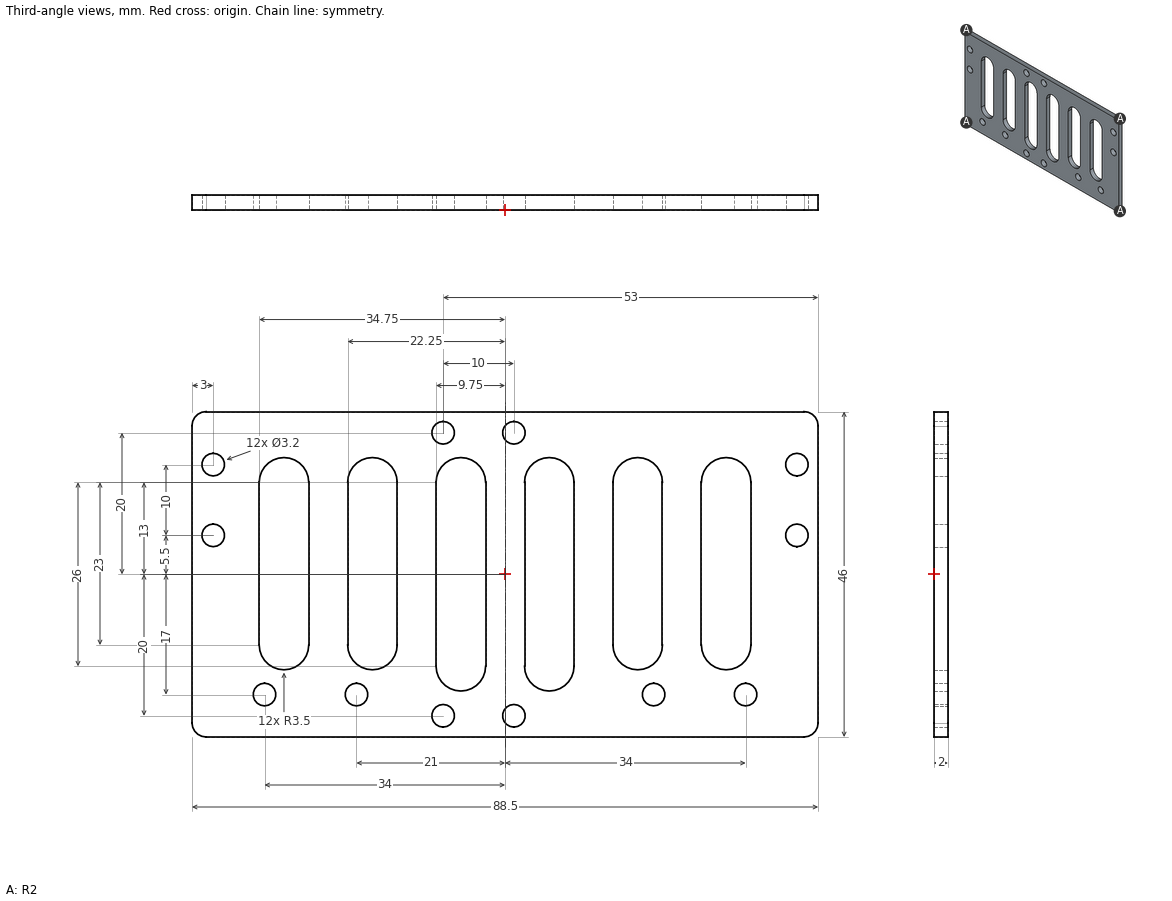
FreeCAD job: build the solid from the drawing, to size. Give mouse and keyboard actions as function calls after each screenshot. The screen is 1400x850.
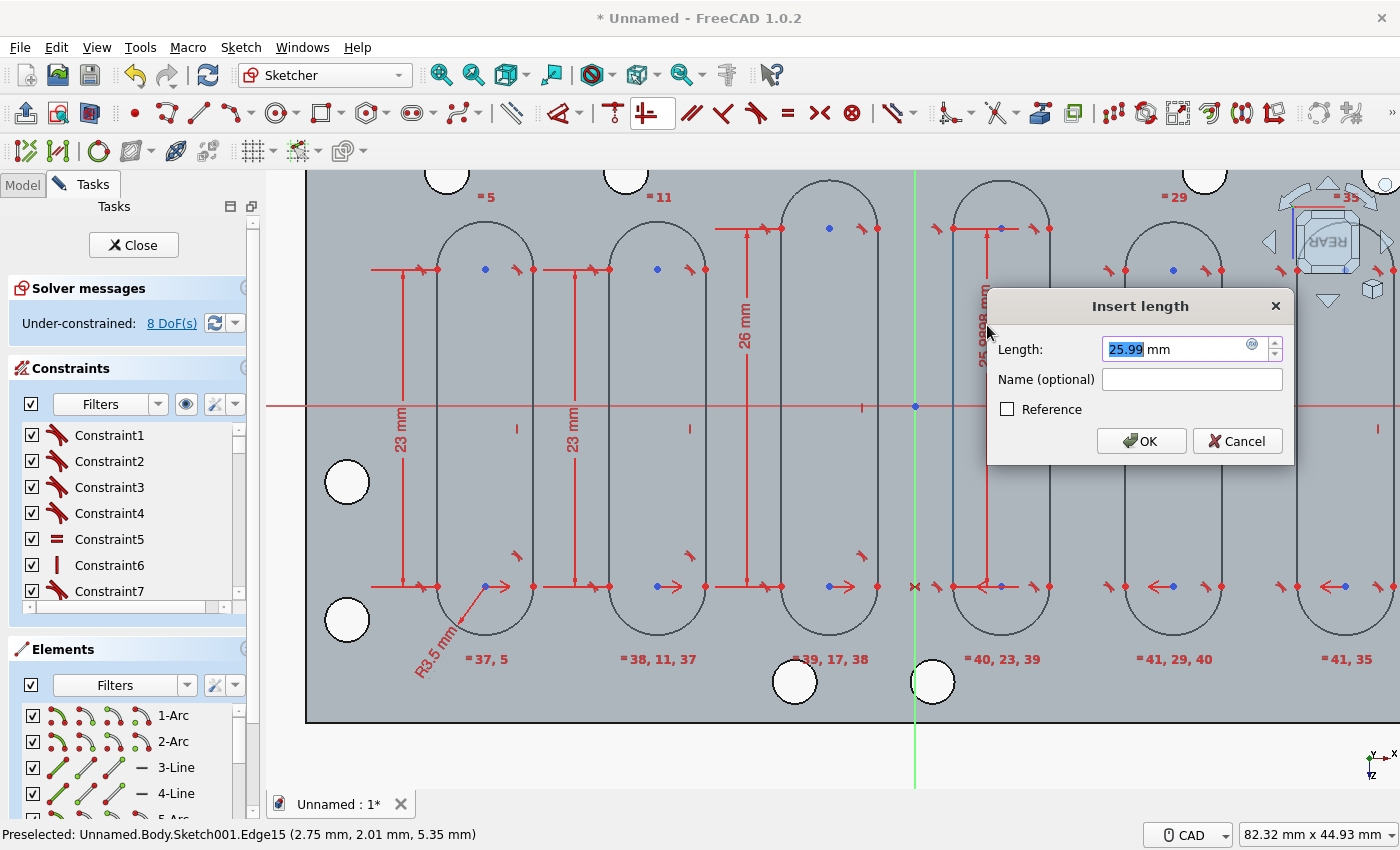
text(26)
key(Return)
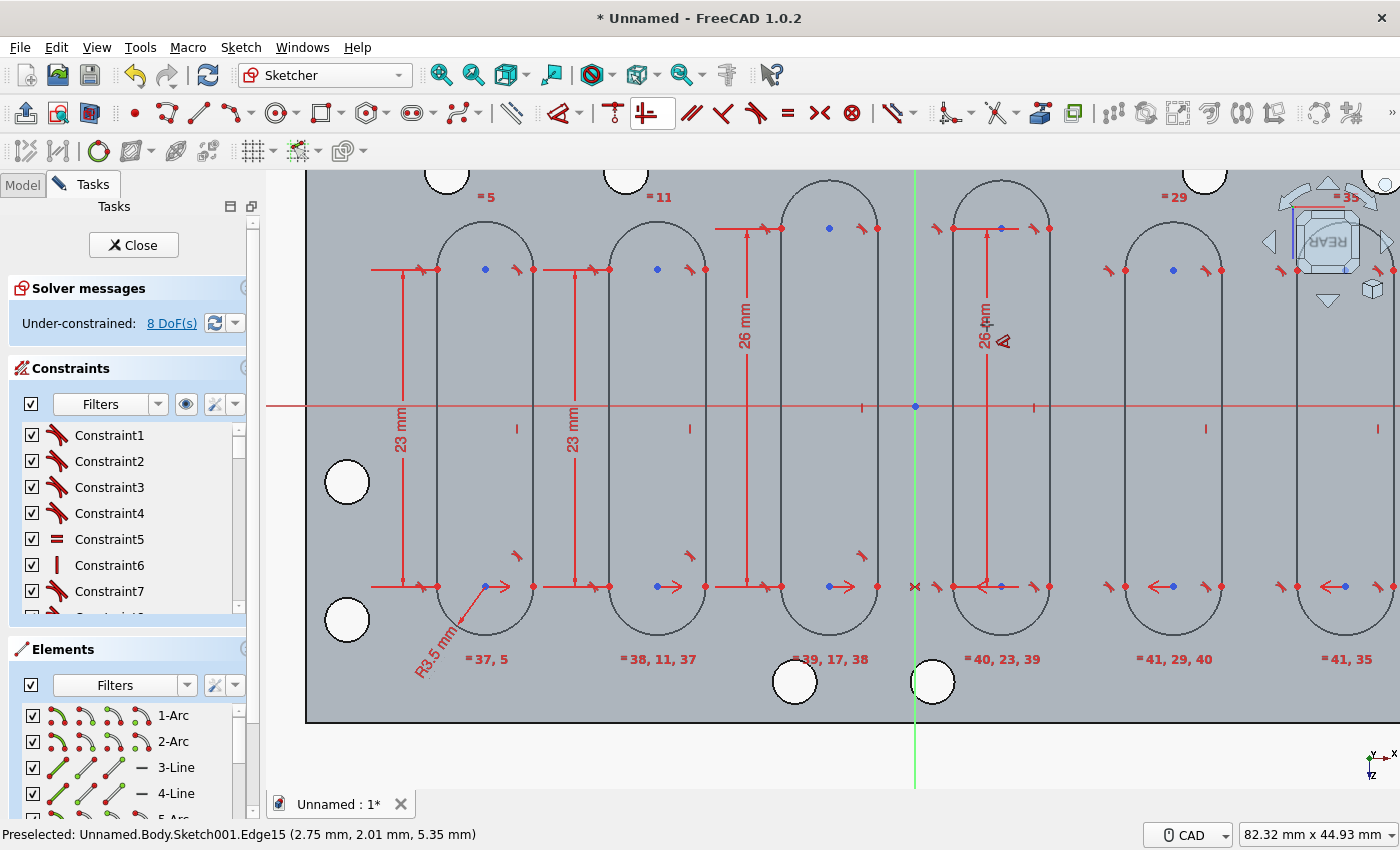
click(1125, 492)
click(1159, 429)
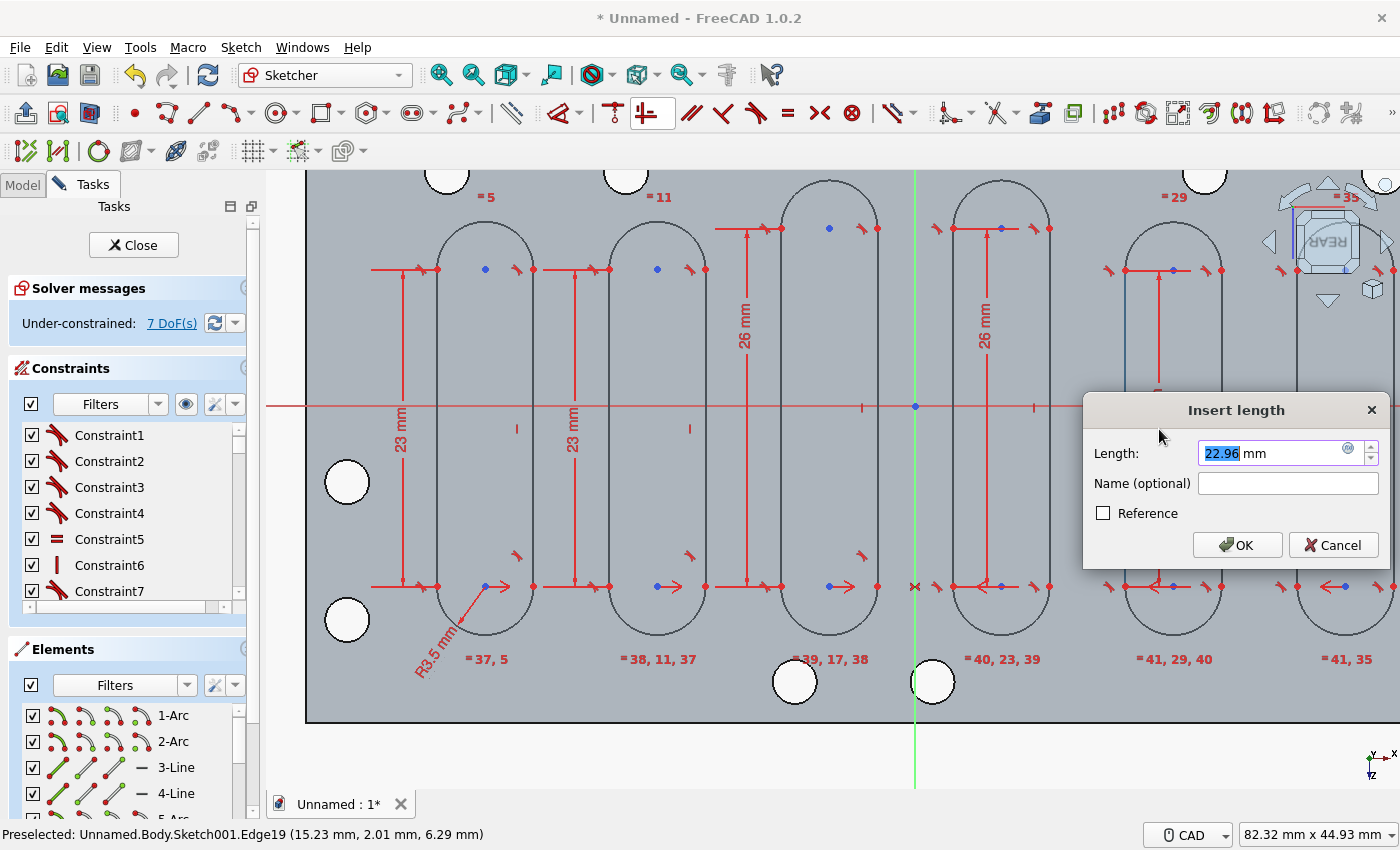
text(23)
key(Return)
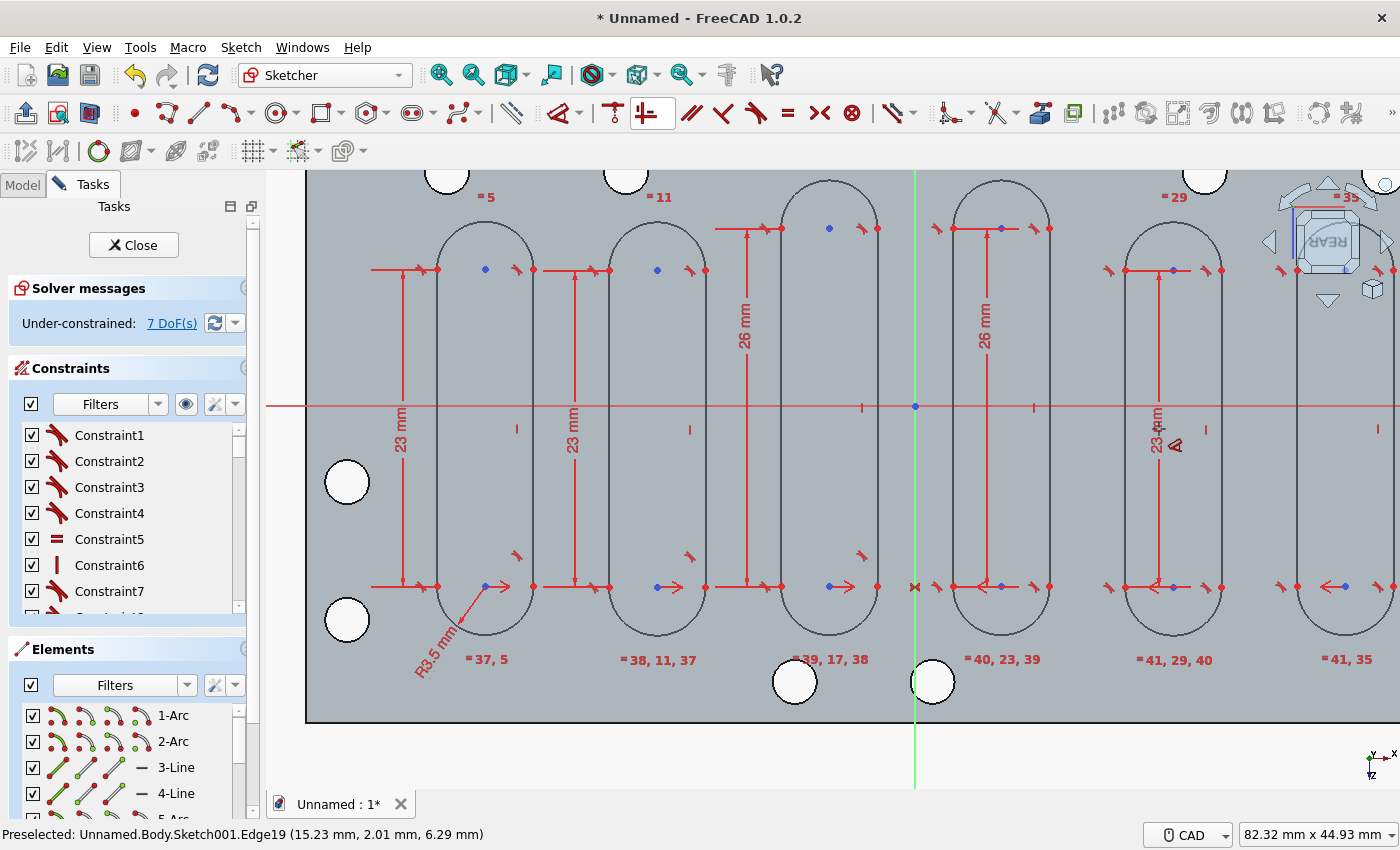
scroll(458, 628, down, 2)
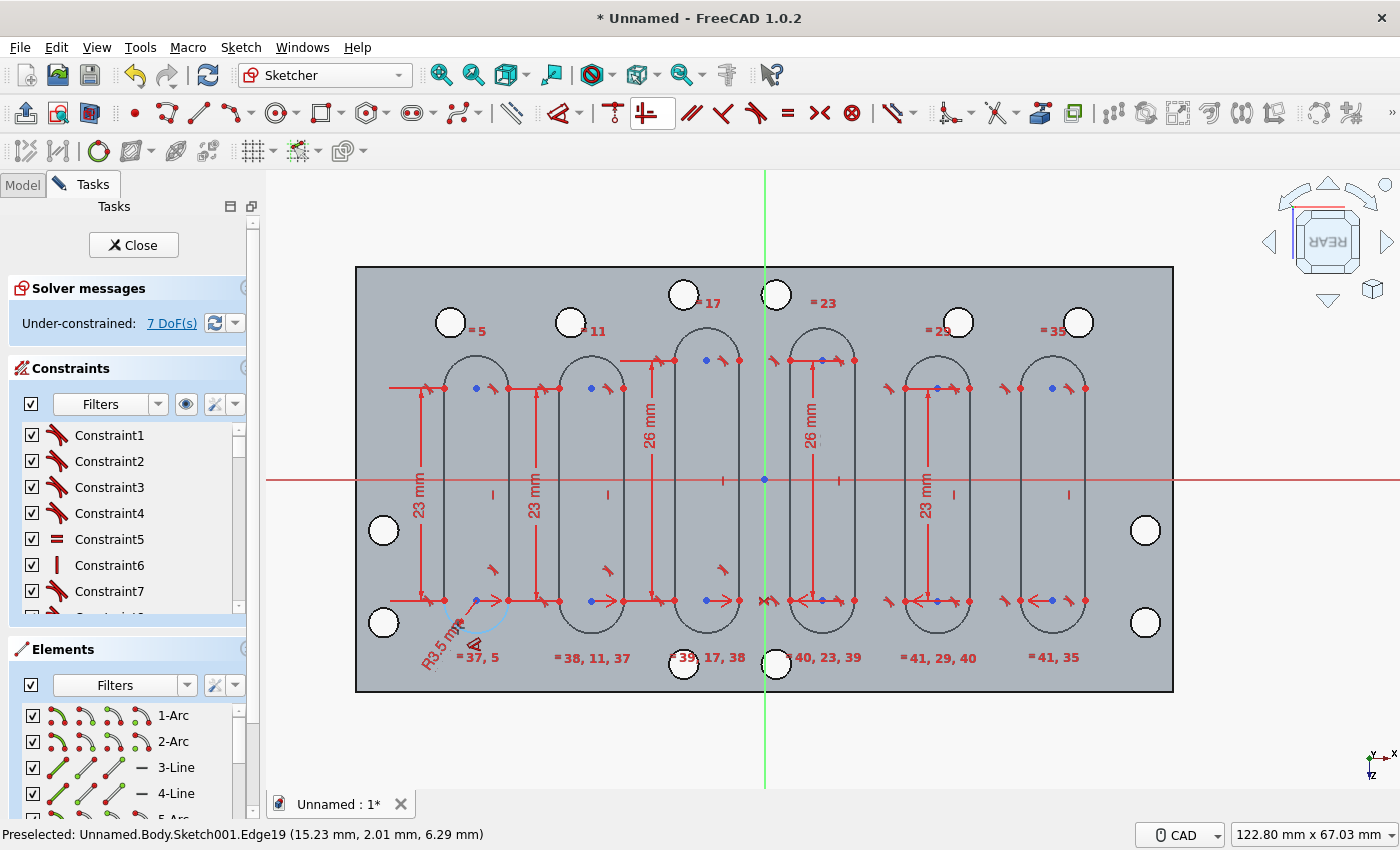
click(1021, 537)
click(1055, 495)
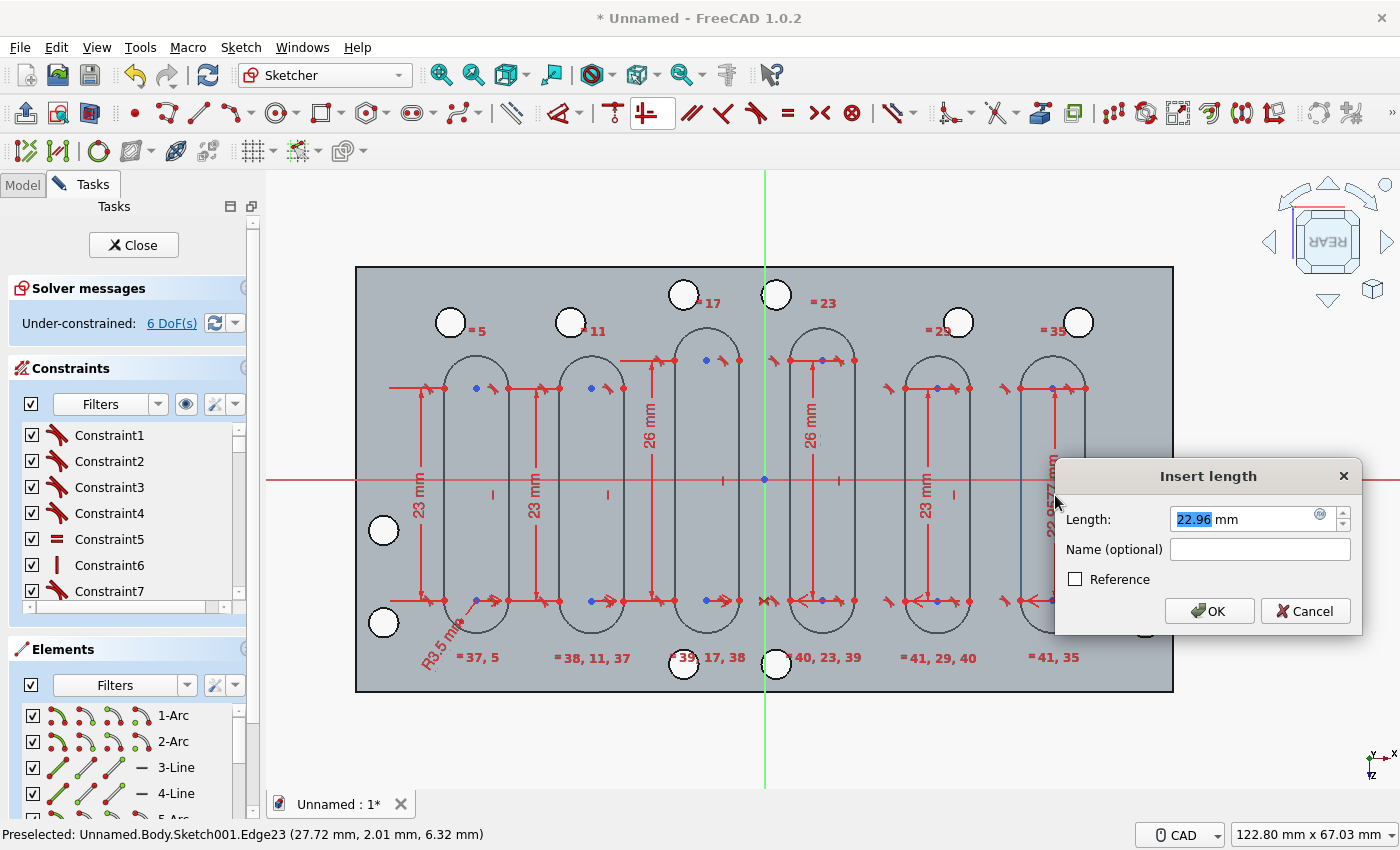
text(23)
key(Return)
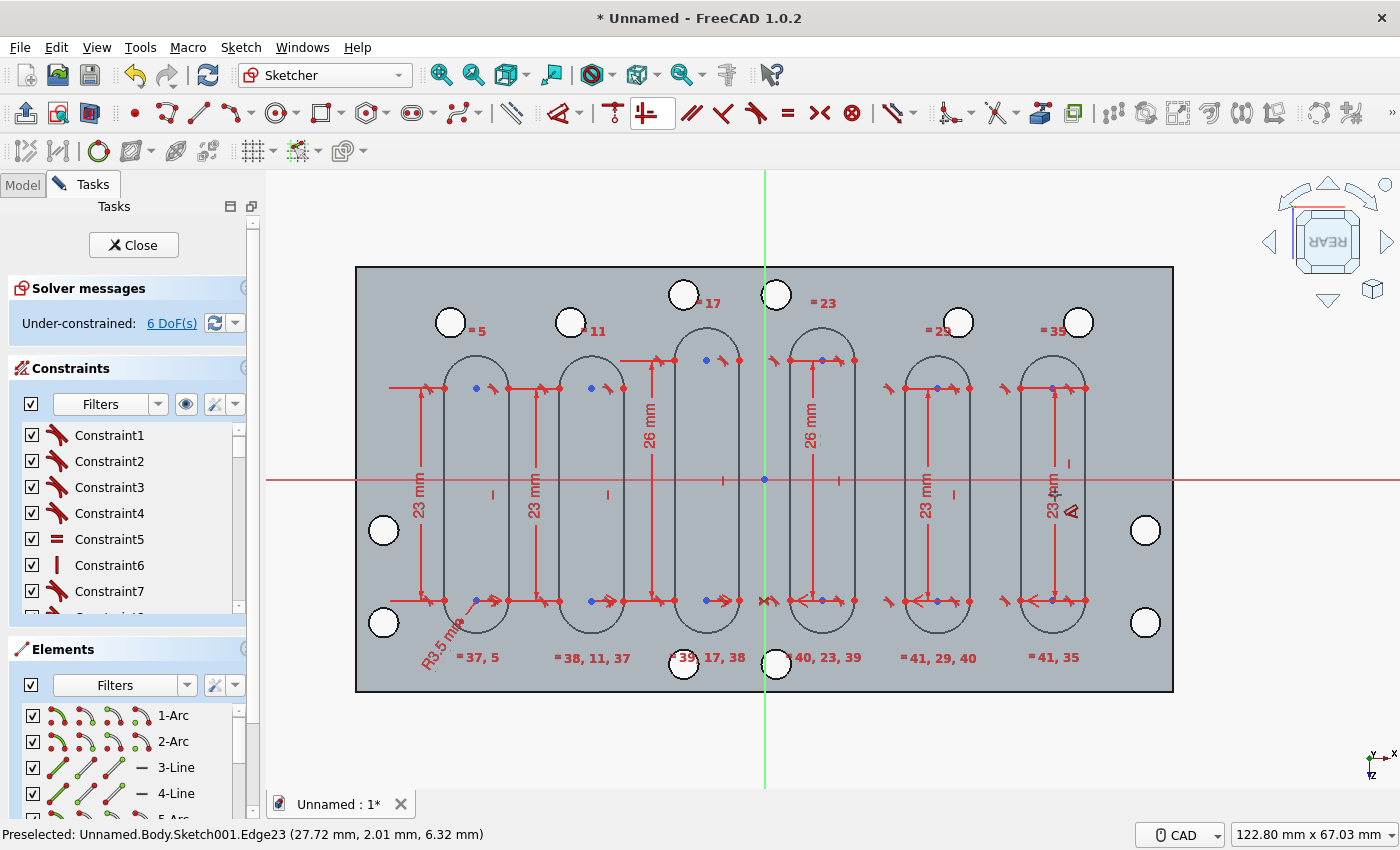
click(444, 601)
click(410, 540)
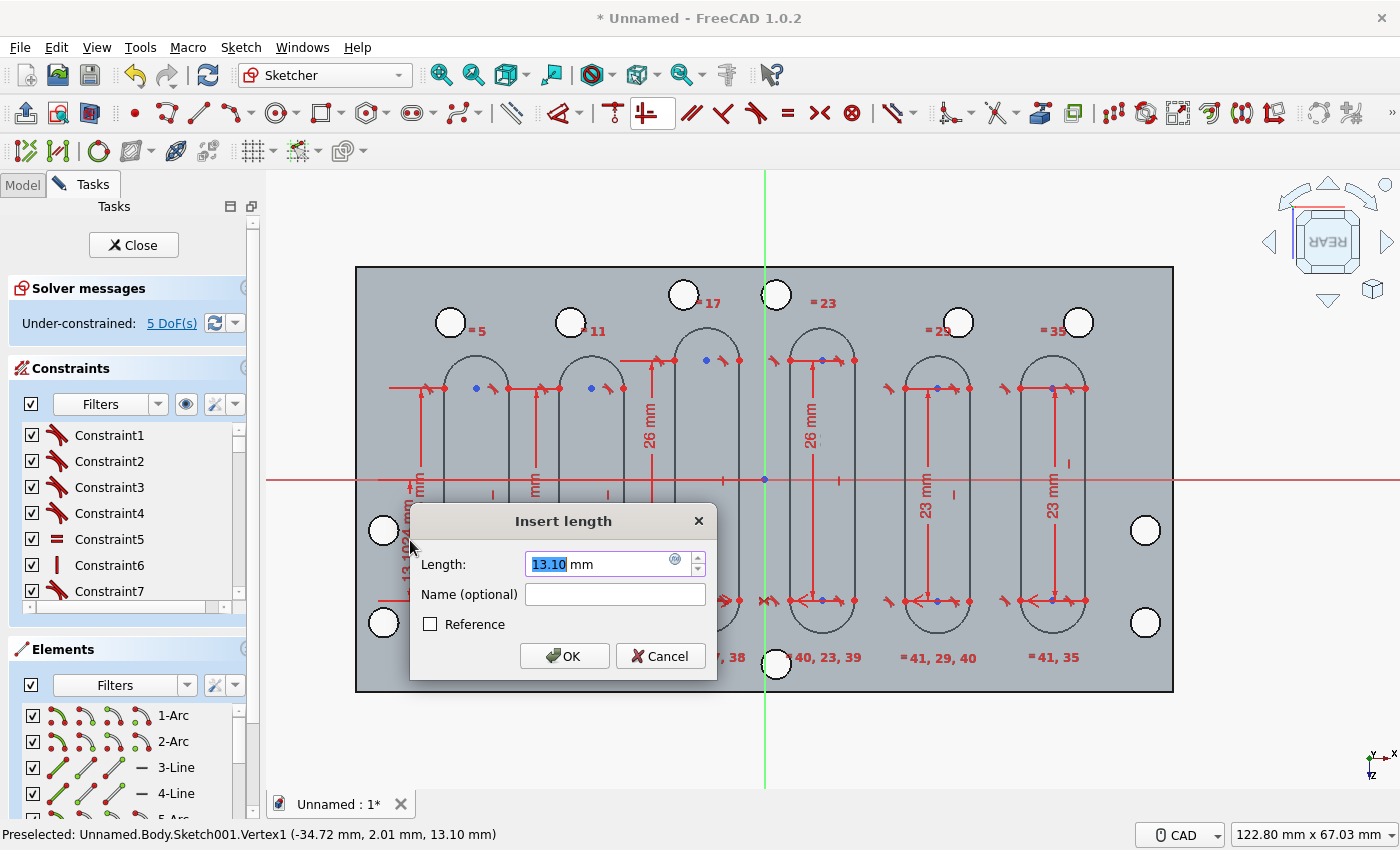
text(13)
key(Return)